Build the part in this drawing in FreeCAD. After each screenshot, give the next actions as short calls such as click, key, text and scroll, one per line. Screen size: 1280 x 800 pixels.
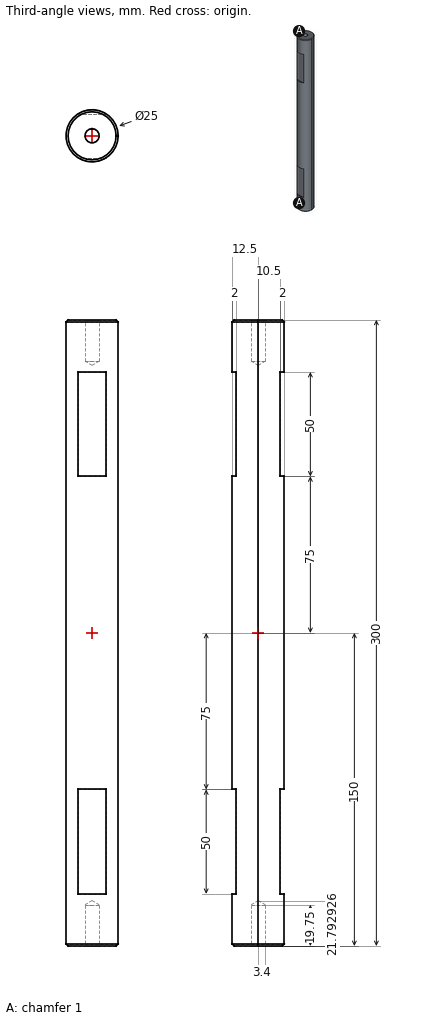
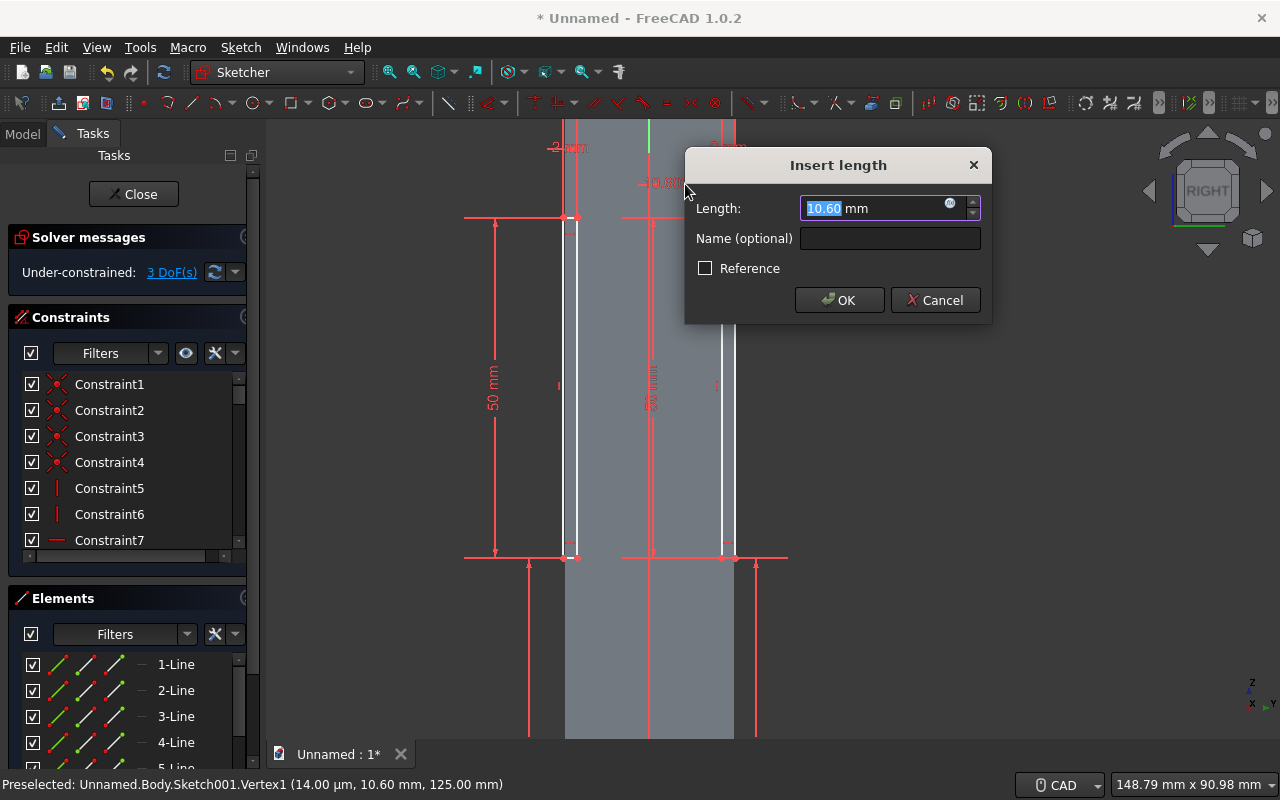
text(10.5)
key(Return)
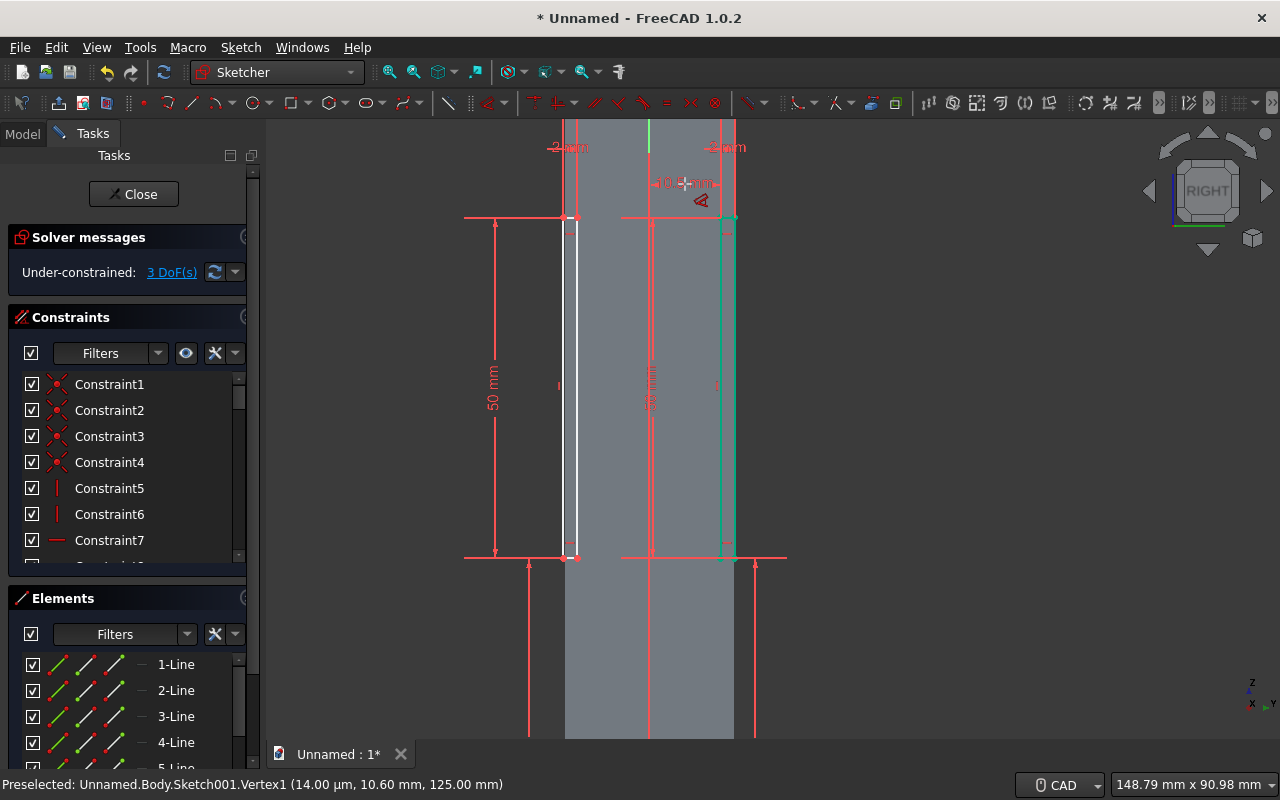
click(563, 218)
click(606, 184)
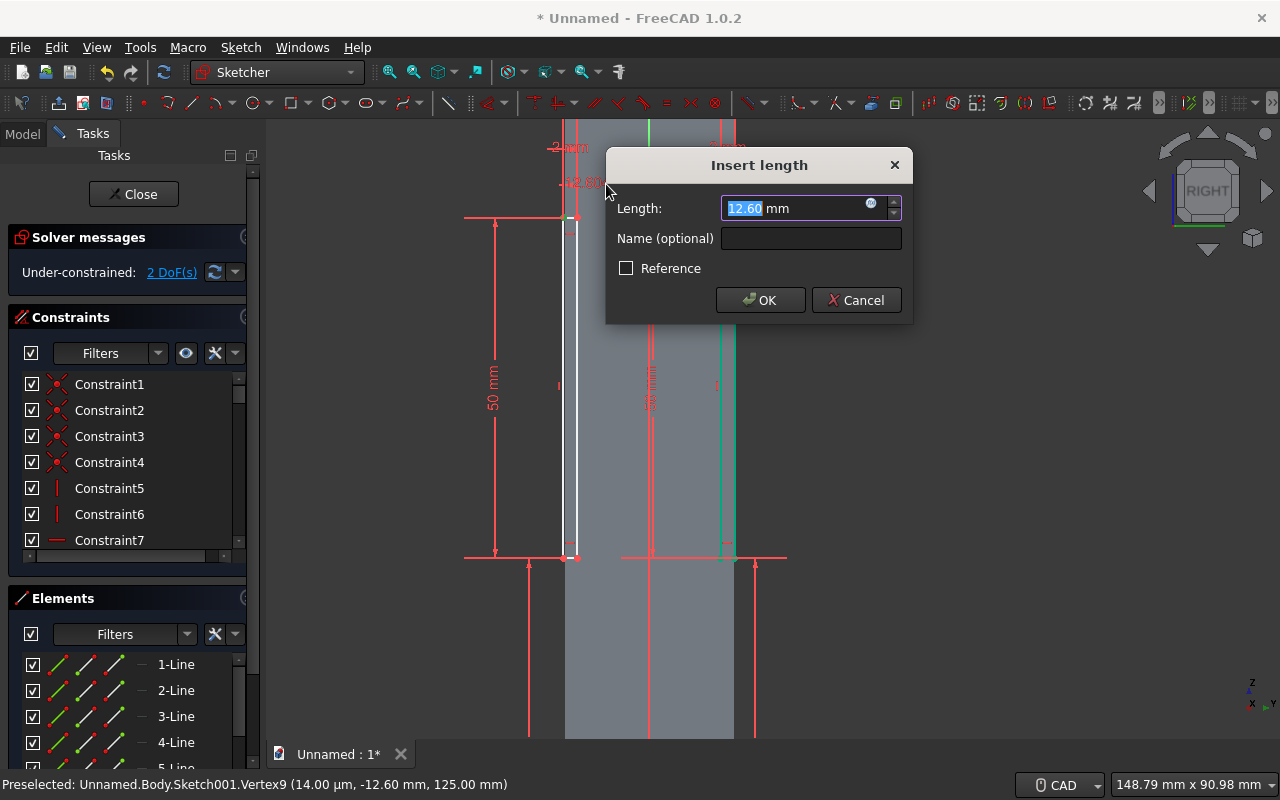
text(12.5)
key(Return)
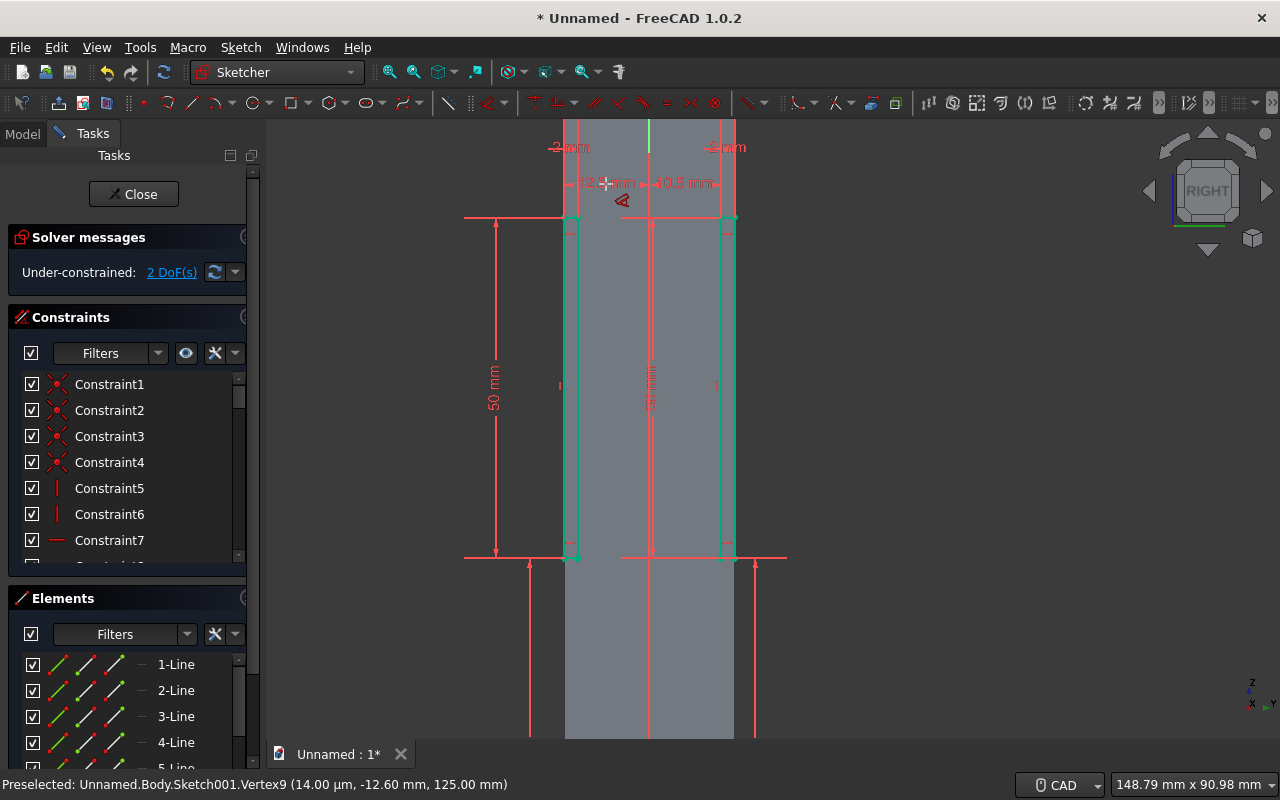
scroll(723, 219, down, 7)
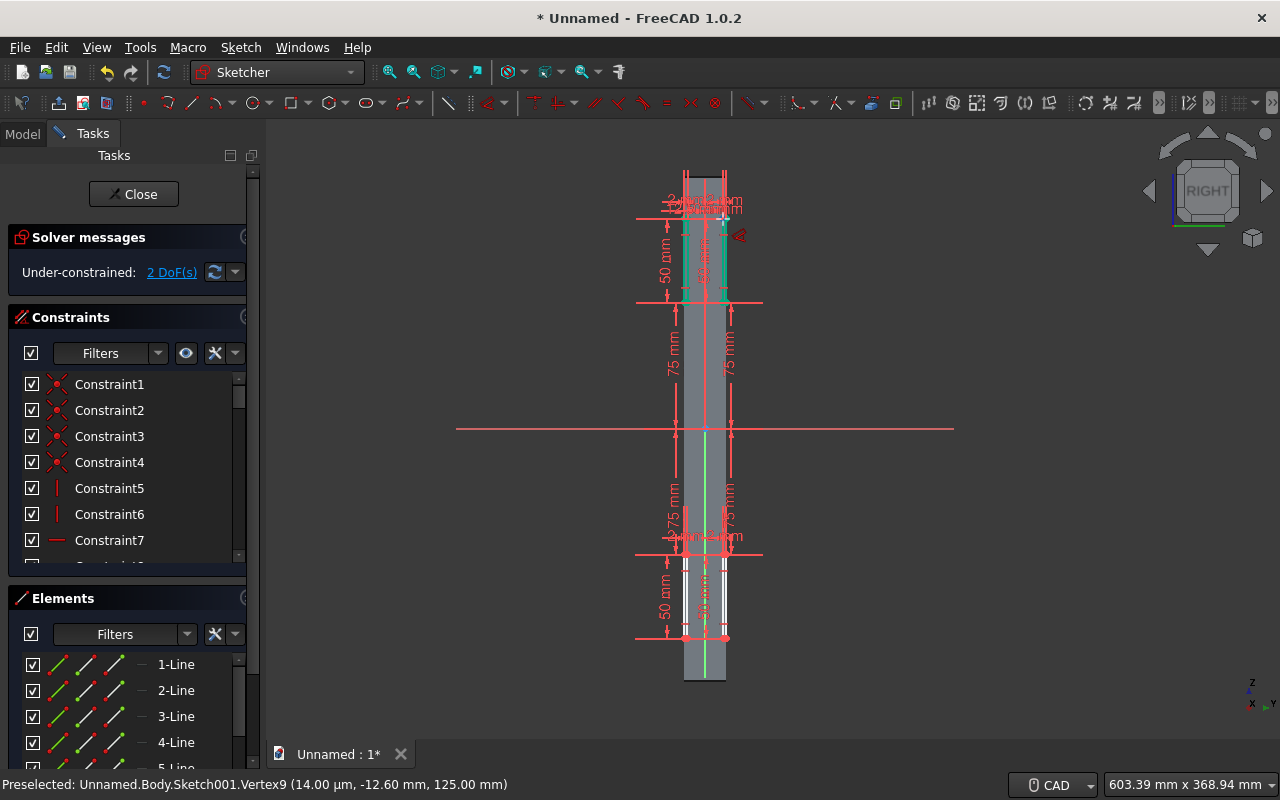
scroll(684, 555, up, 7)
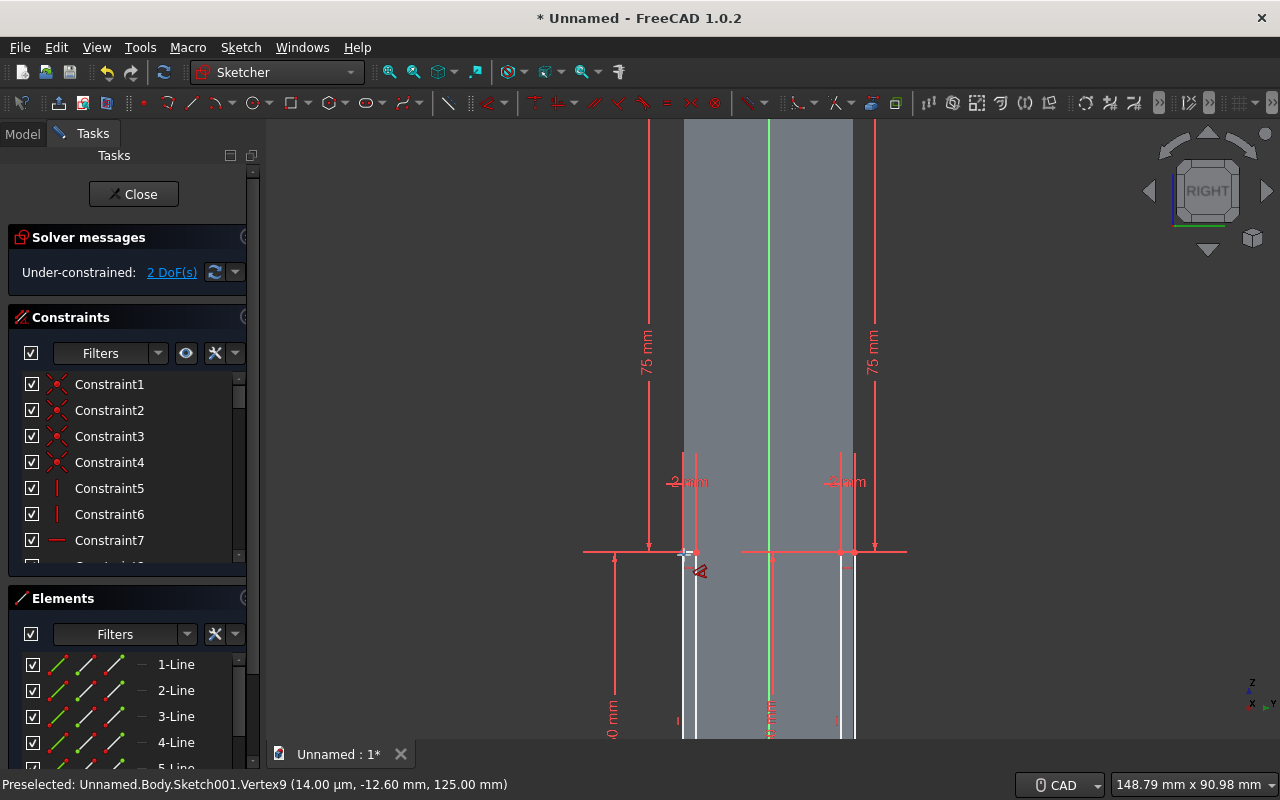
click(683, 552)
click(726, 586)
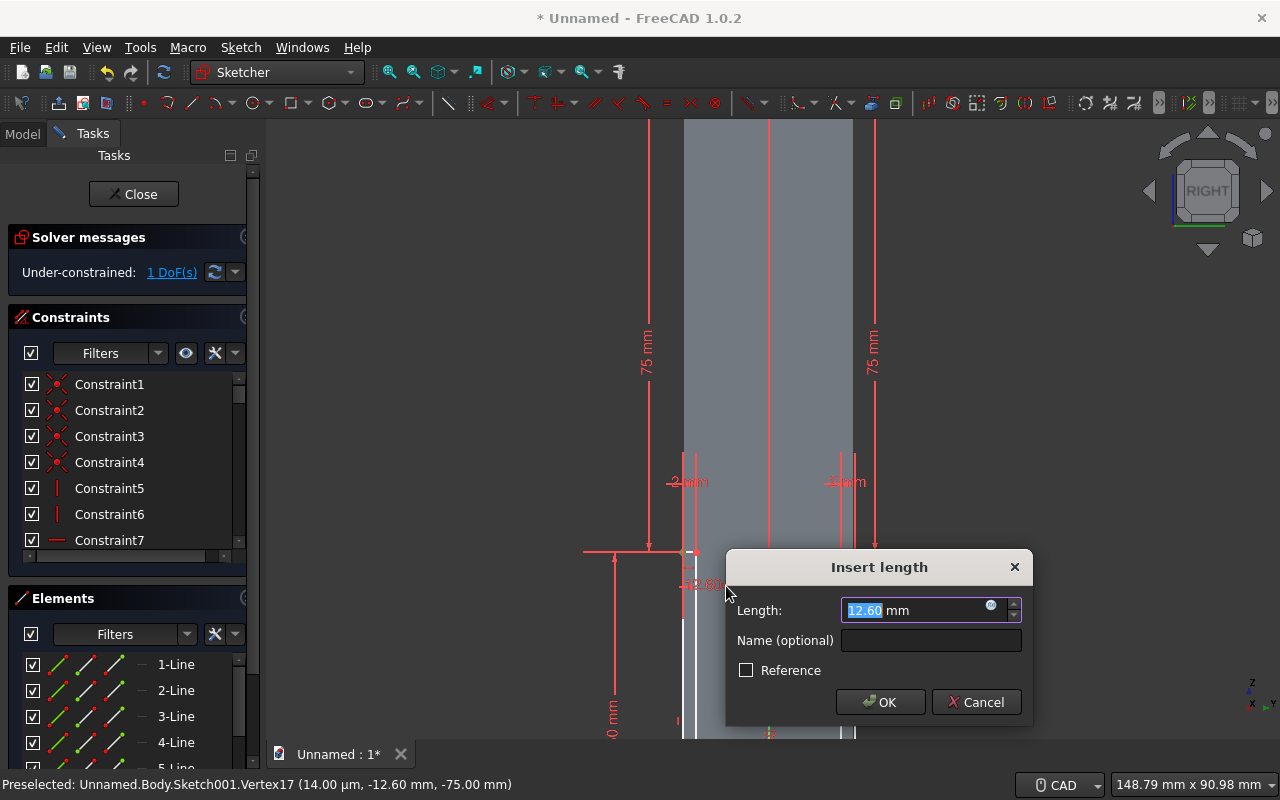
text(12.5)
key(Return)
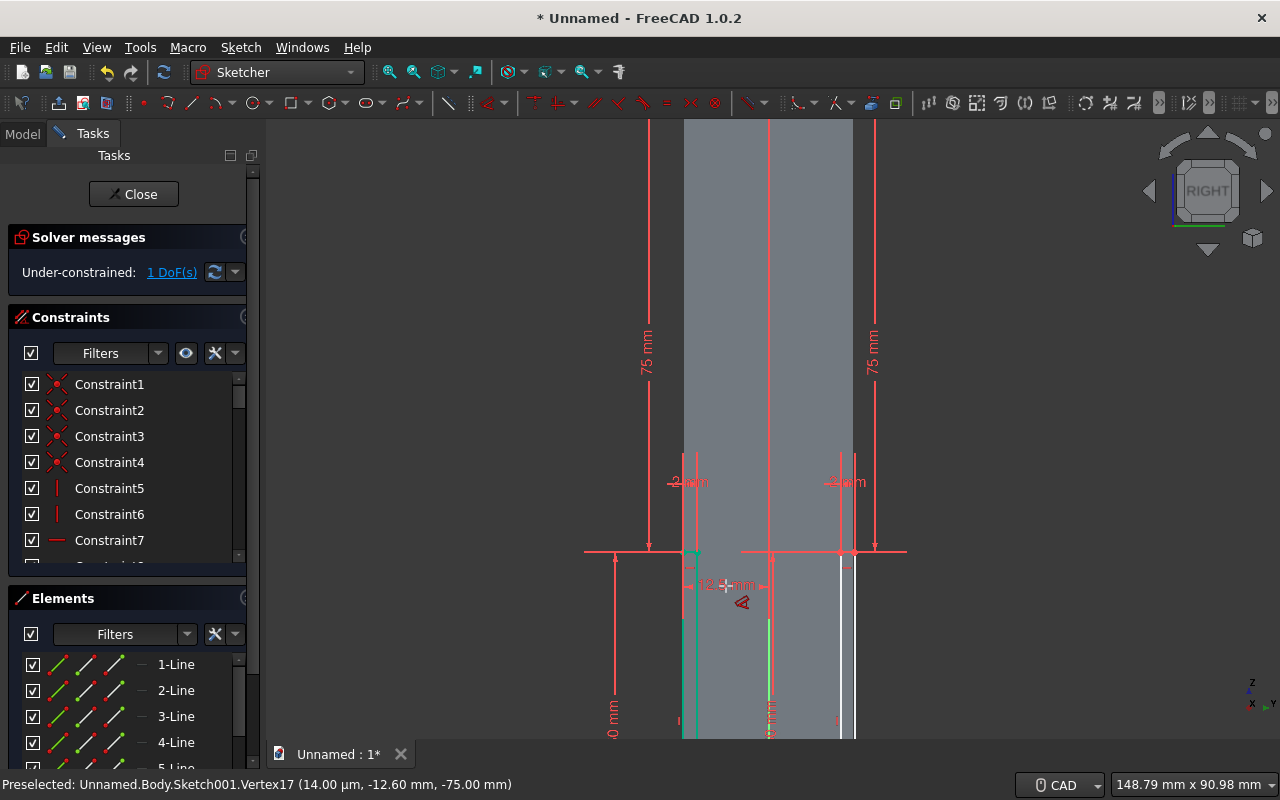
click(841, 552)
click(805, 586)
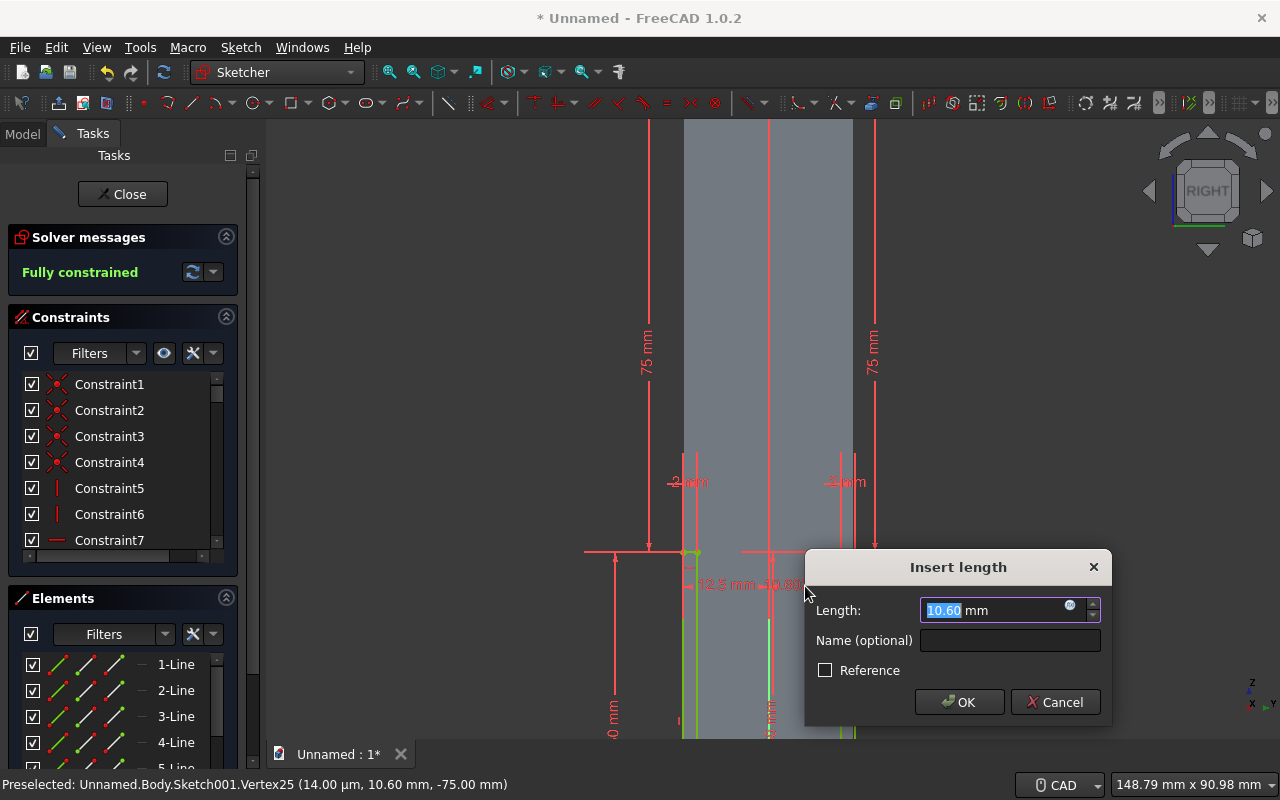
text(10.5)
key(Return)
key(Escape)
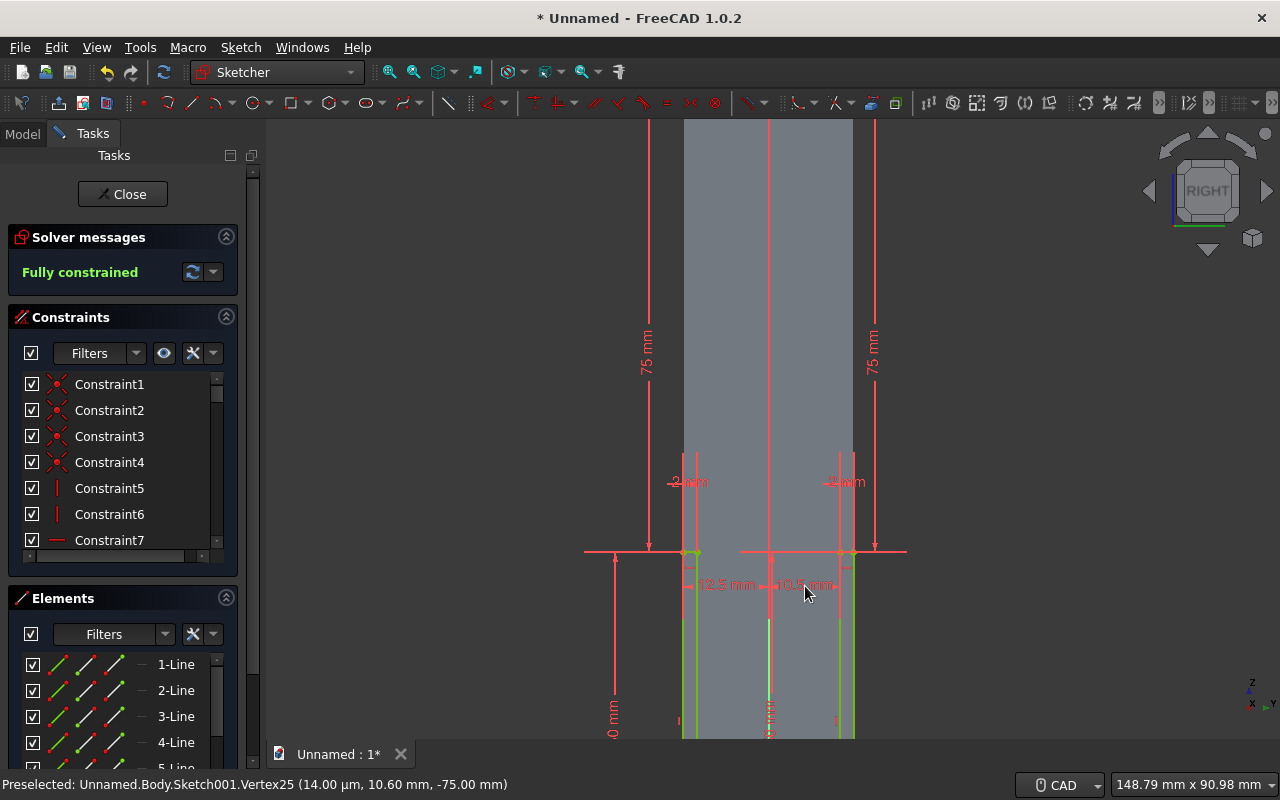
click(123, 194)